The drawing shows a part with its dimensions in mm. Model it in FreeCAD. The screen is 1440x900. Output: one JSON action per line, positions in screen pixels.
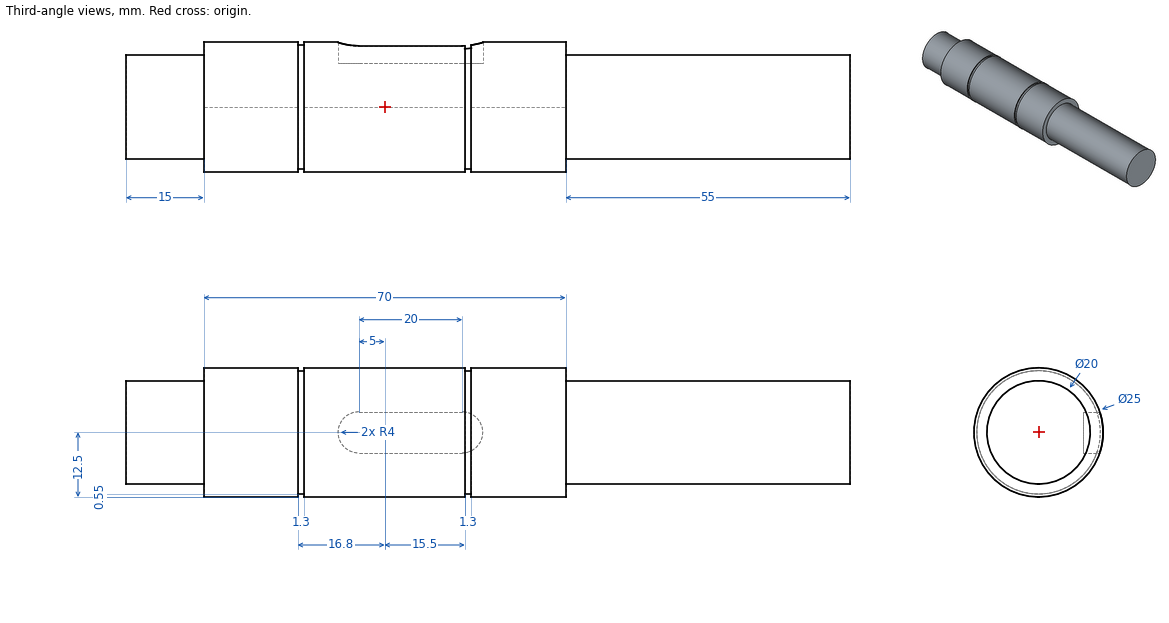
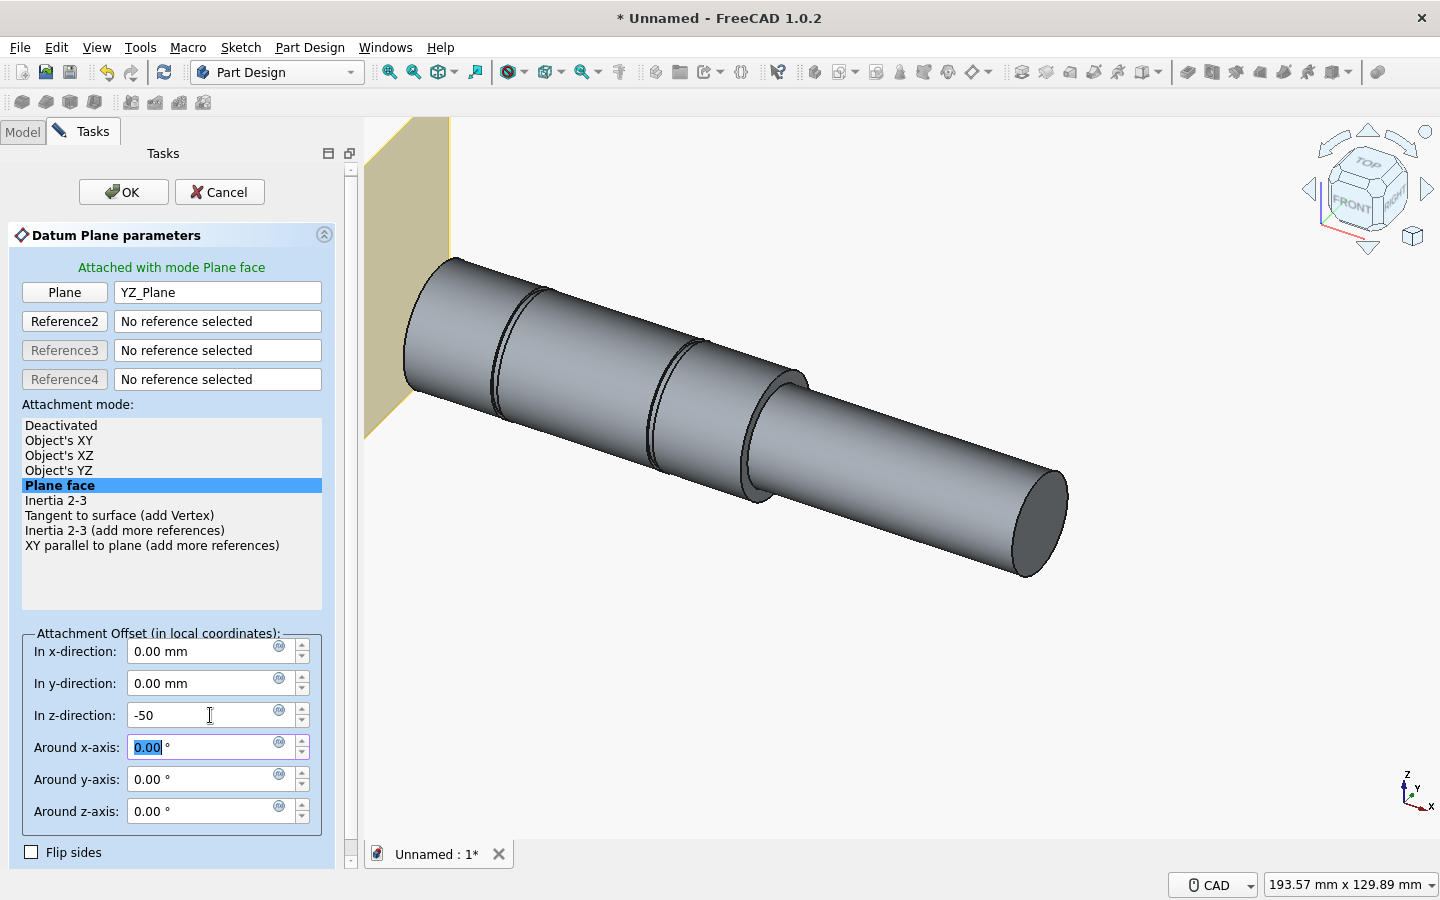
{"action": "left_click", "coordinate": [124, 192]}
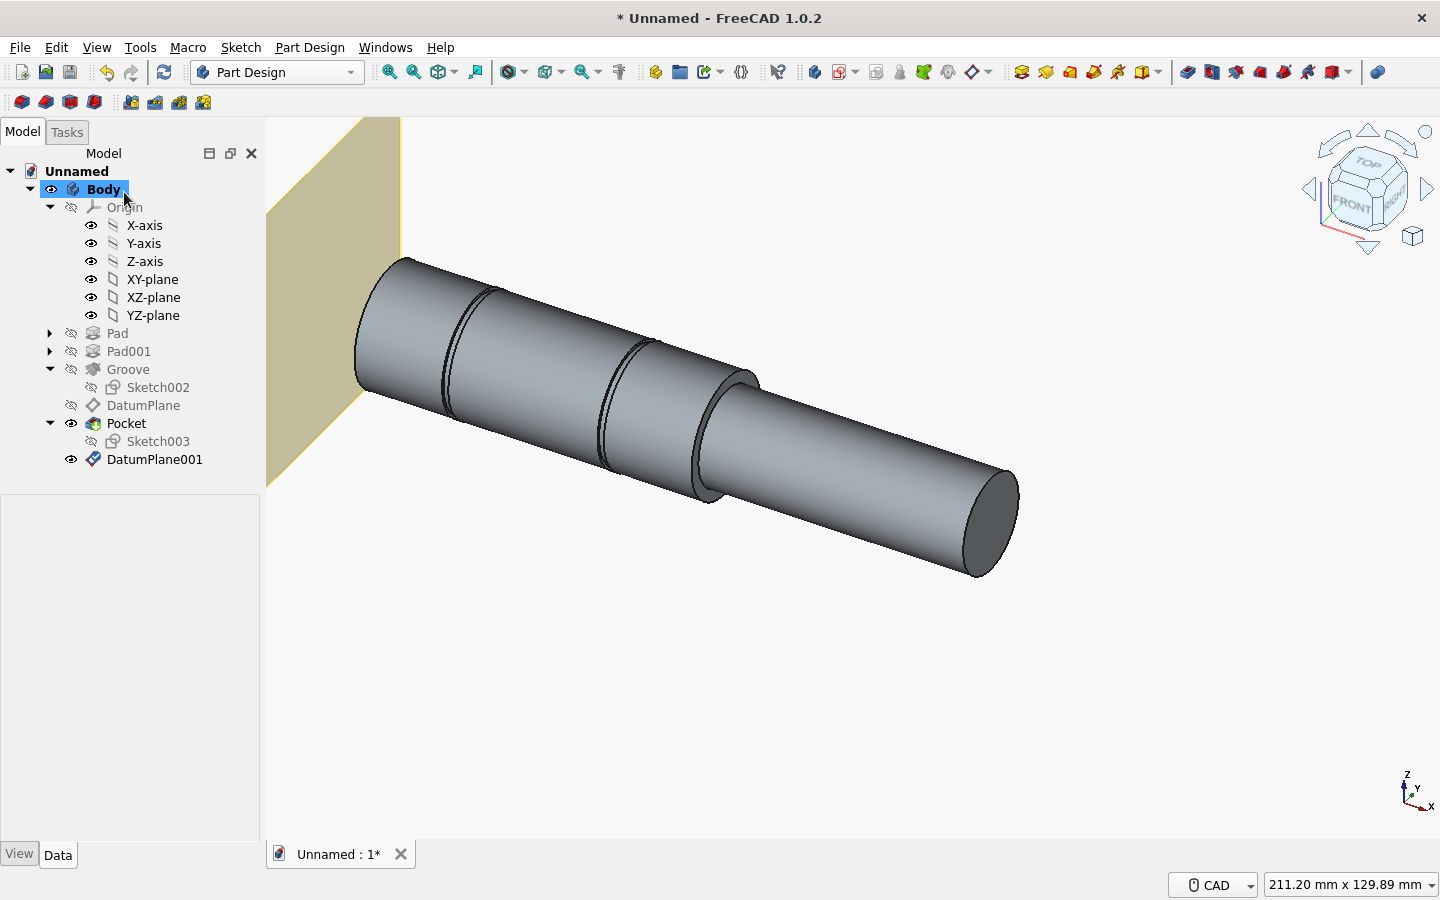
{"action": "left_click", "coordinate": [116, 459]}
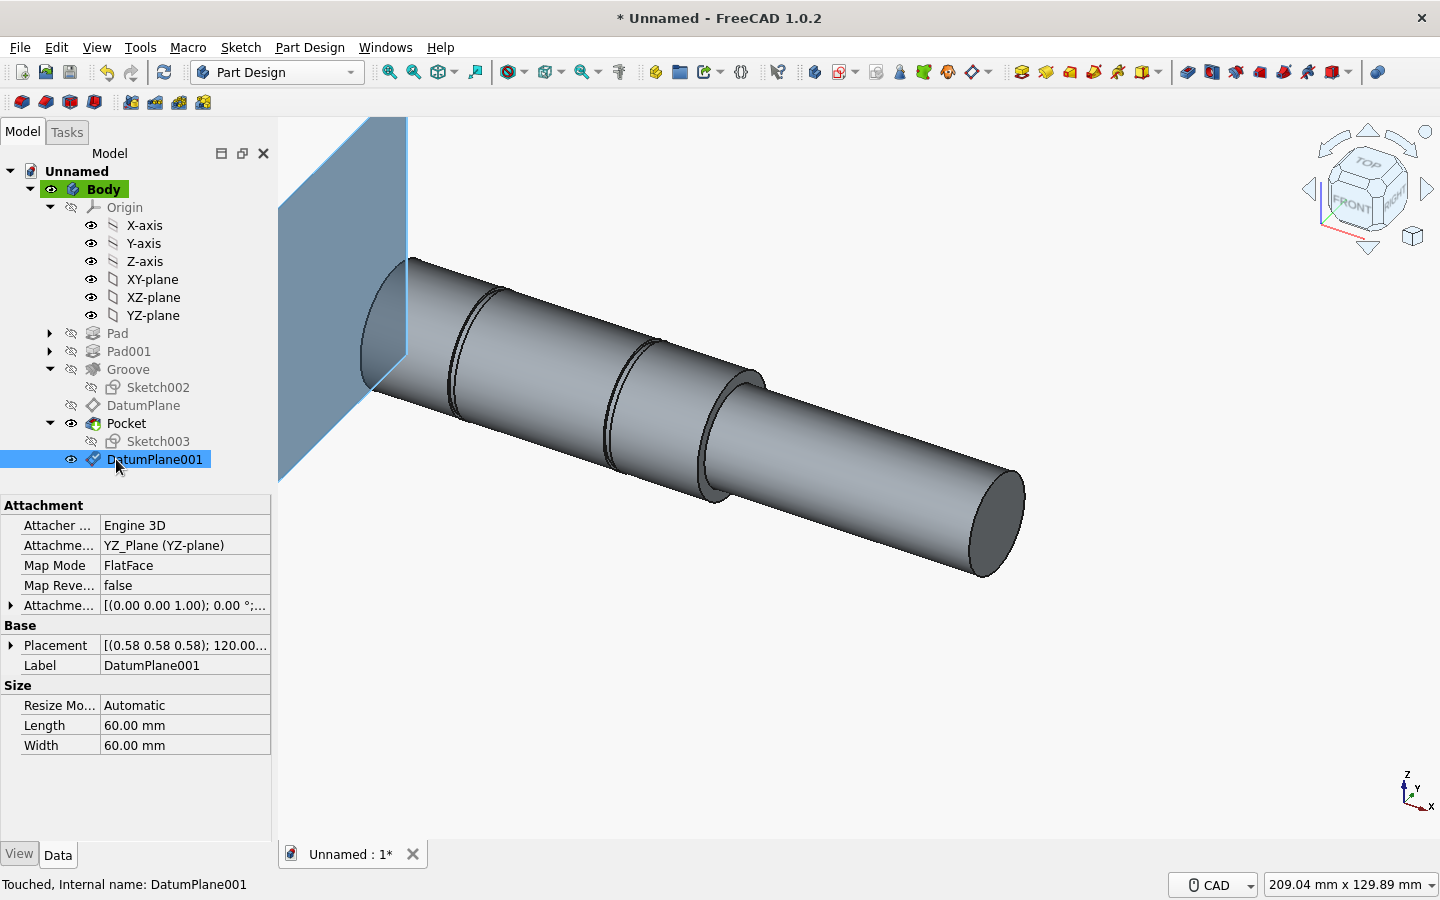
{"action": "left_click", "coordinate": [840, 72]}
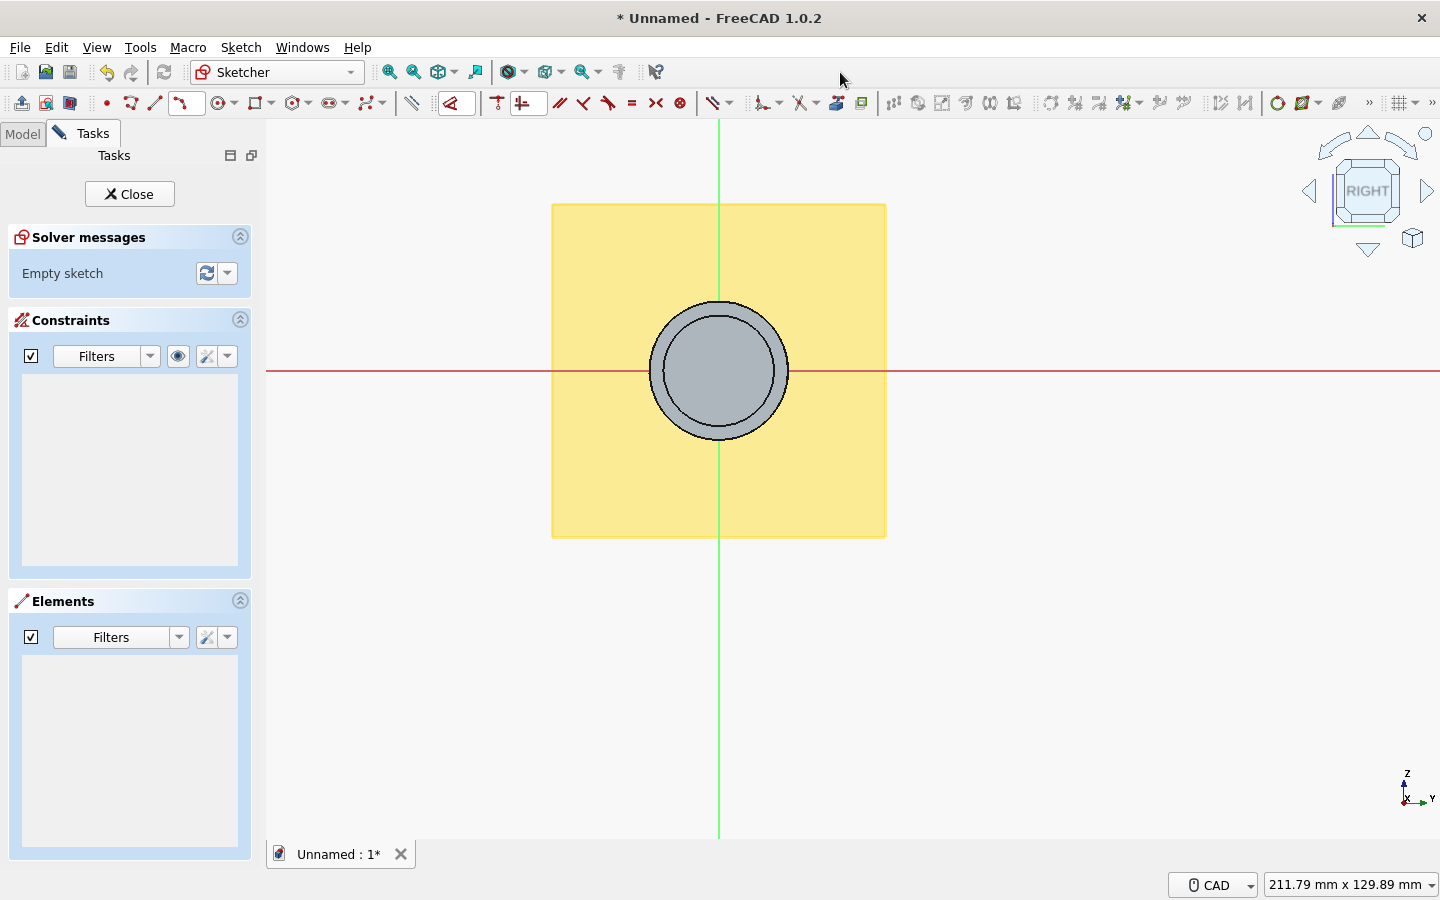
{"action": "key", "text": "q s"}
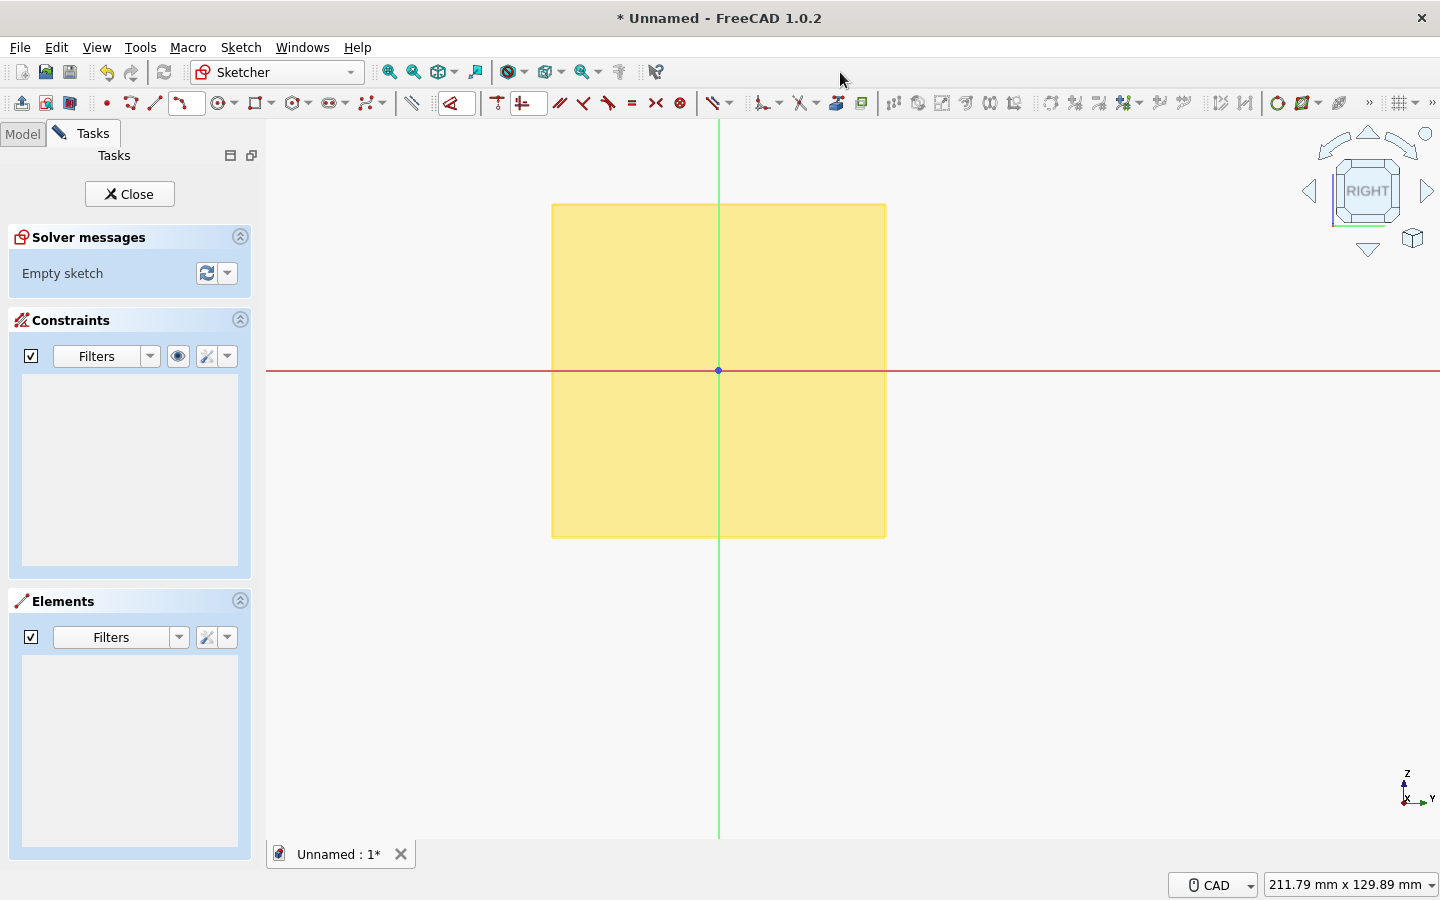
{"action": "scroll", "coordinate": [697, 335], "scroll_direction": "up", "scroll_amount": 7}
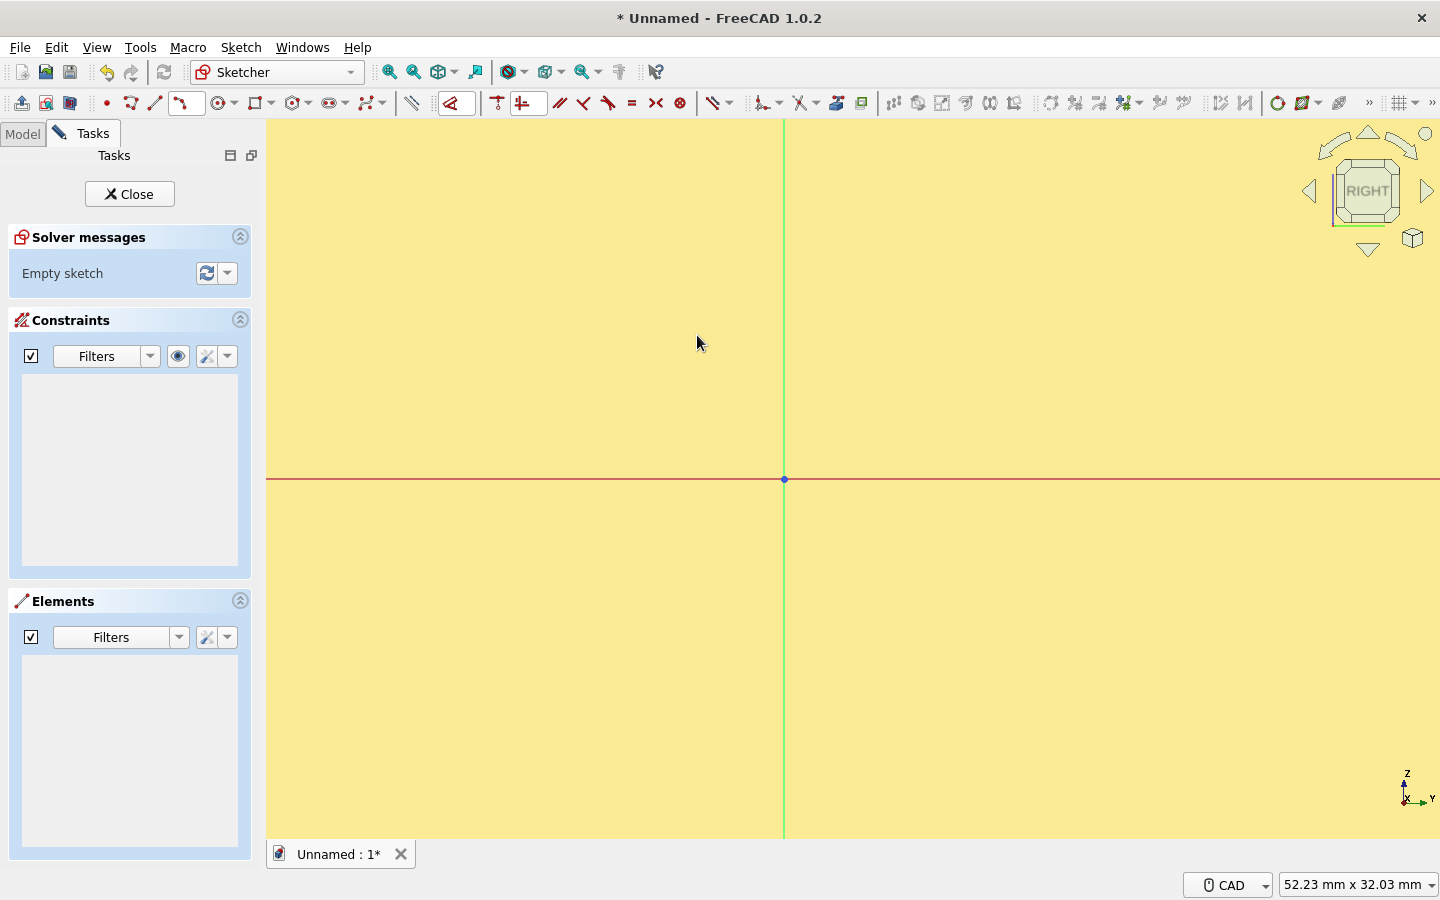
{"action": "key", "text": "g c"}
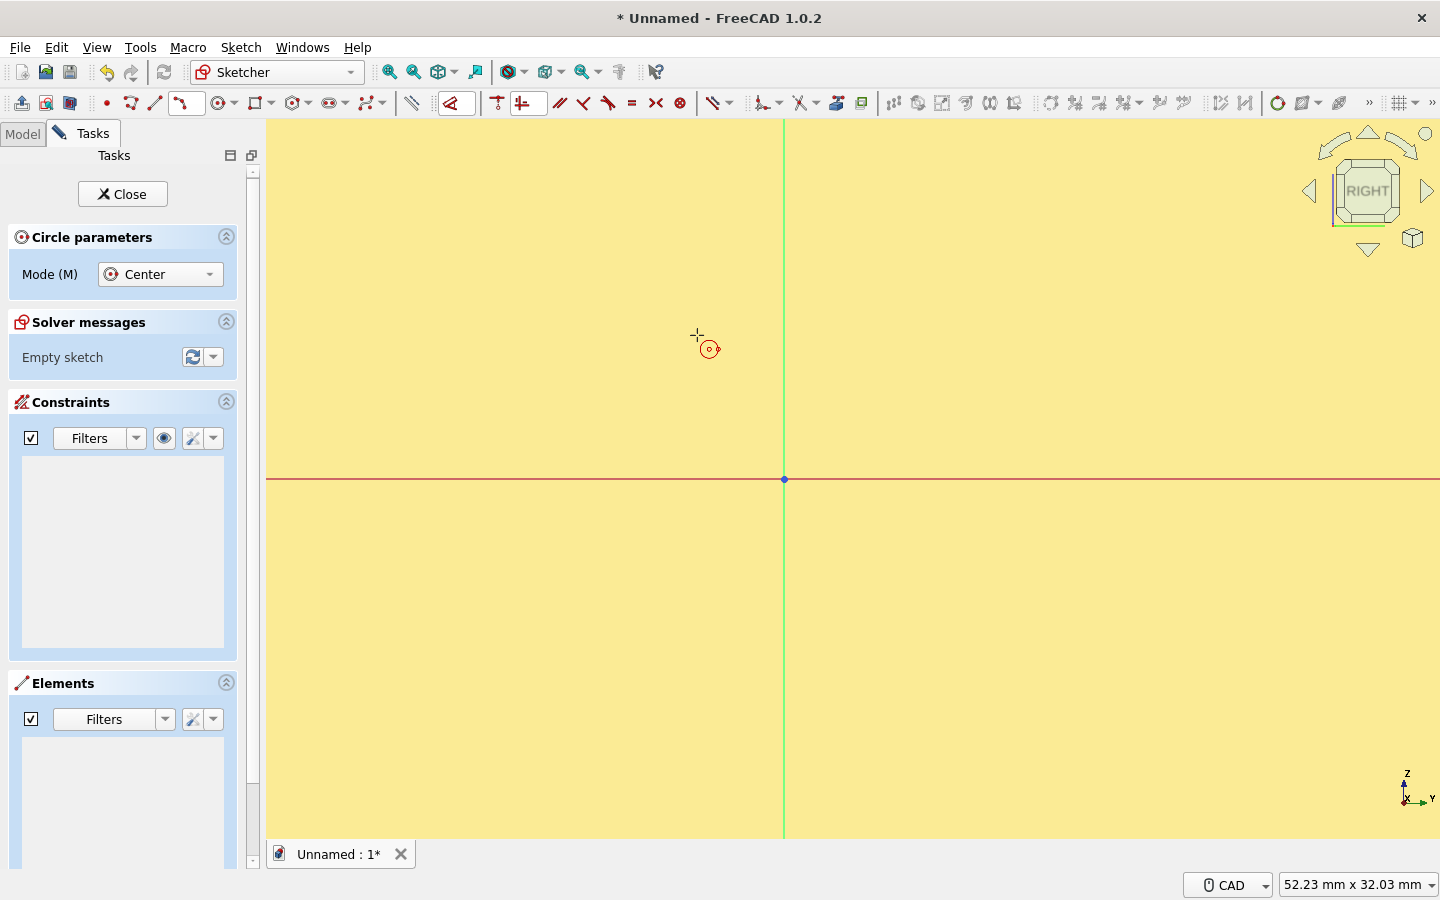
{"action": "left_click", "coordinate": [784, 479]}
{"action": "left_click", "coordinate": [943, 320]}
{"action": "key", "text": "Escape"}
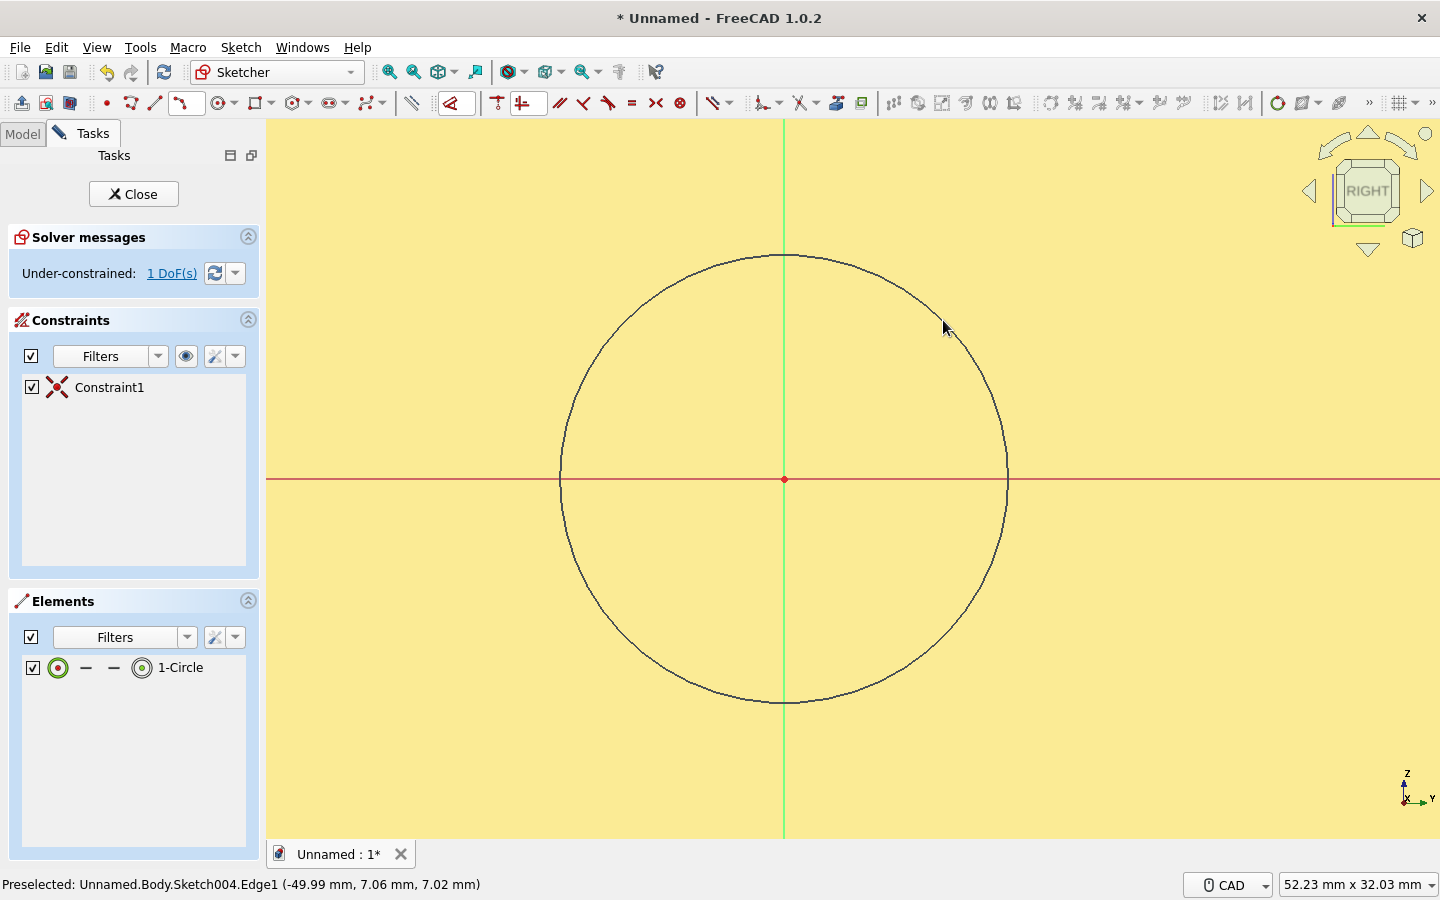
{"action": "left_click", "coordinate": [942, 320]}